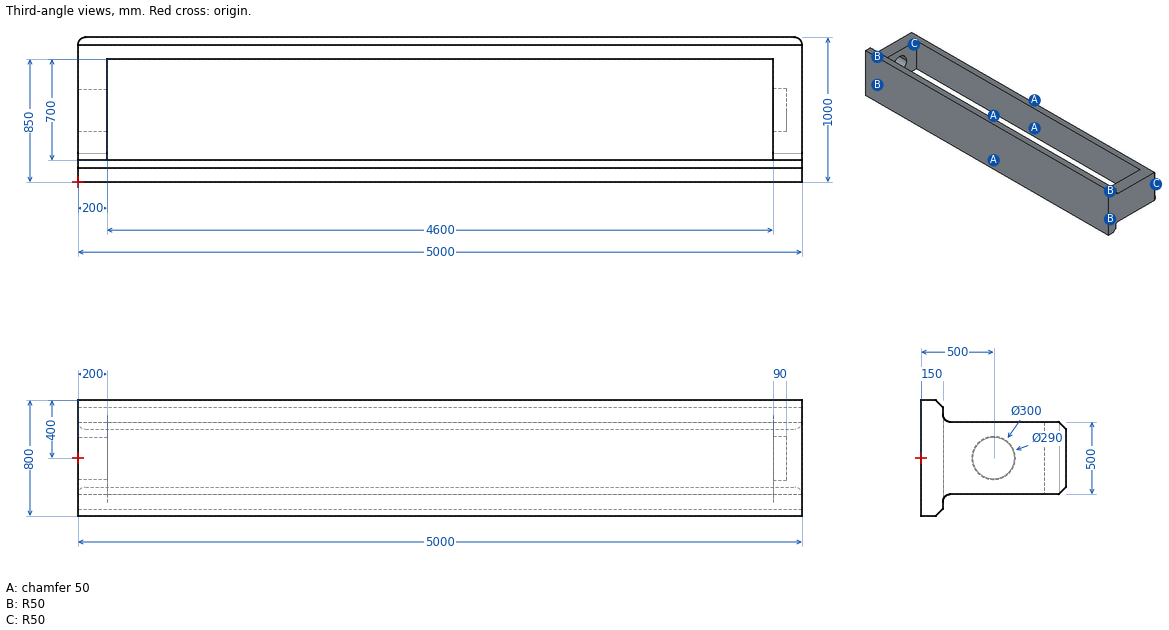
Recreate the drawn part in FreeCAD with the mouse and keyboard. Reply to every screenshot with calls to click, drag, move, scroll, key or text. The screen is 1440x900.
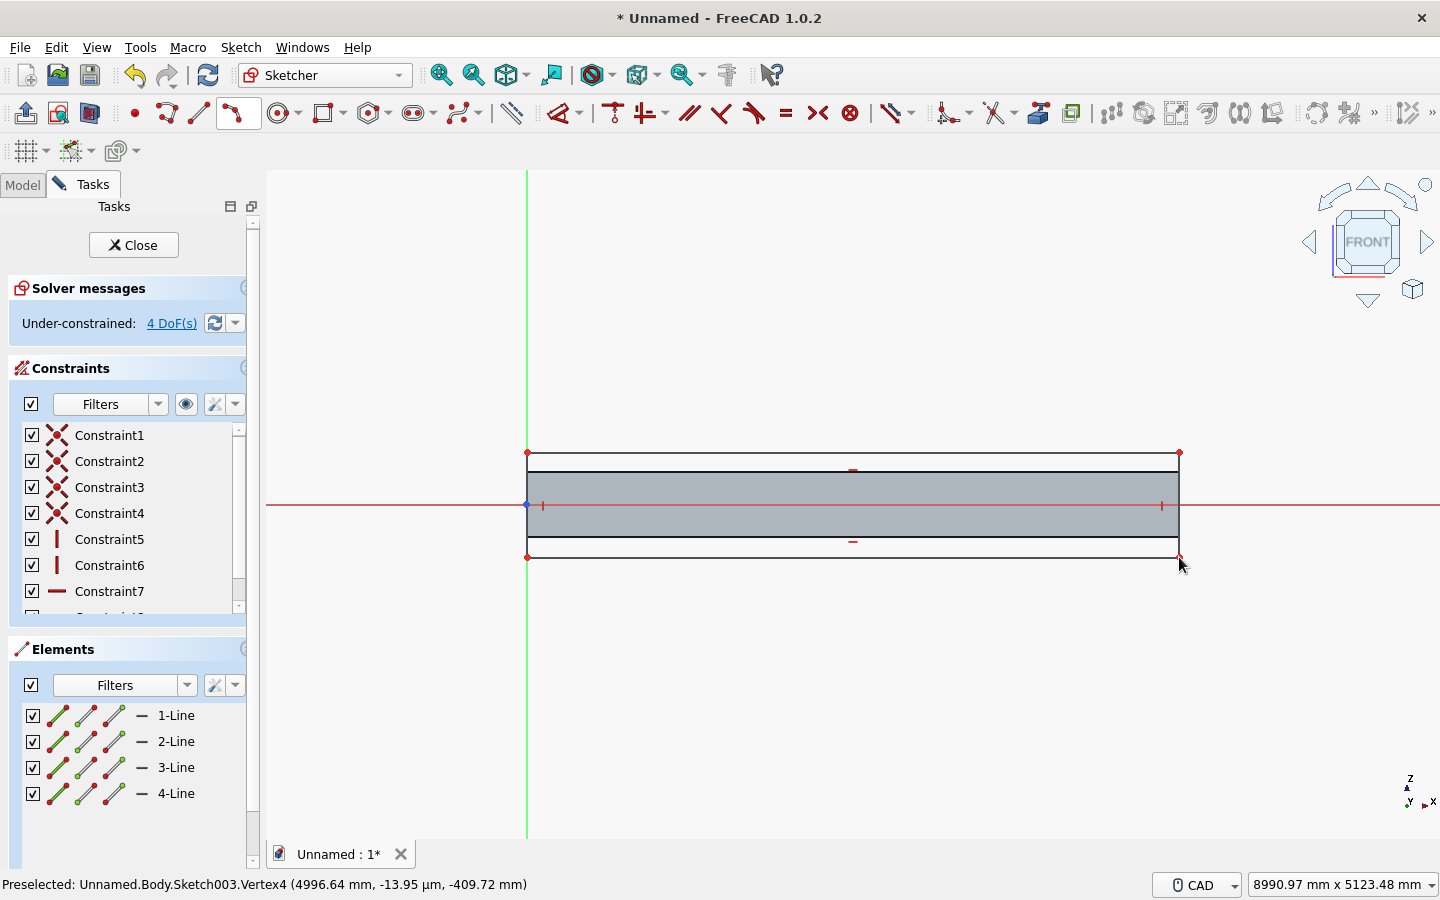
click(527, 453)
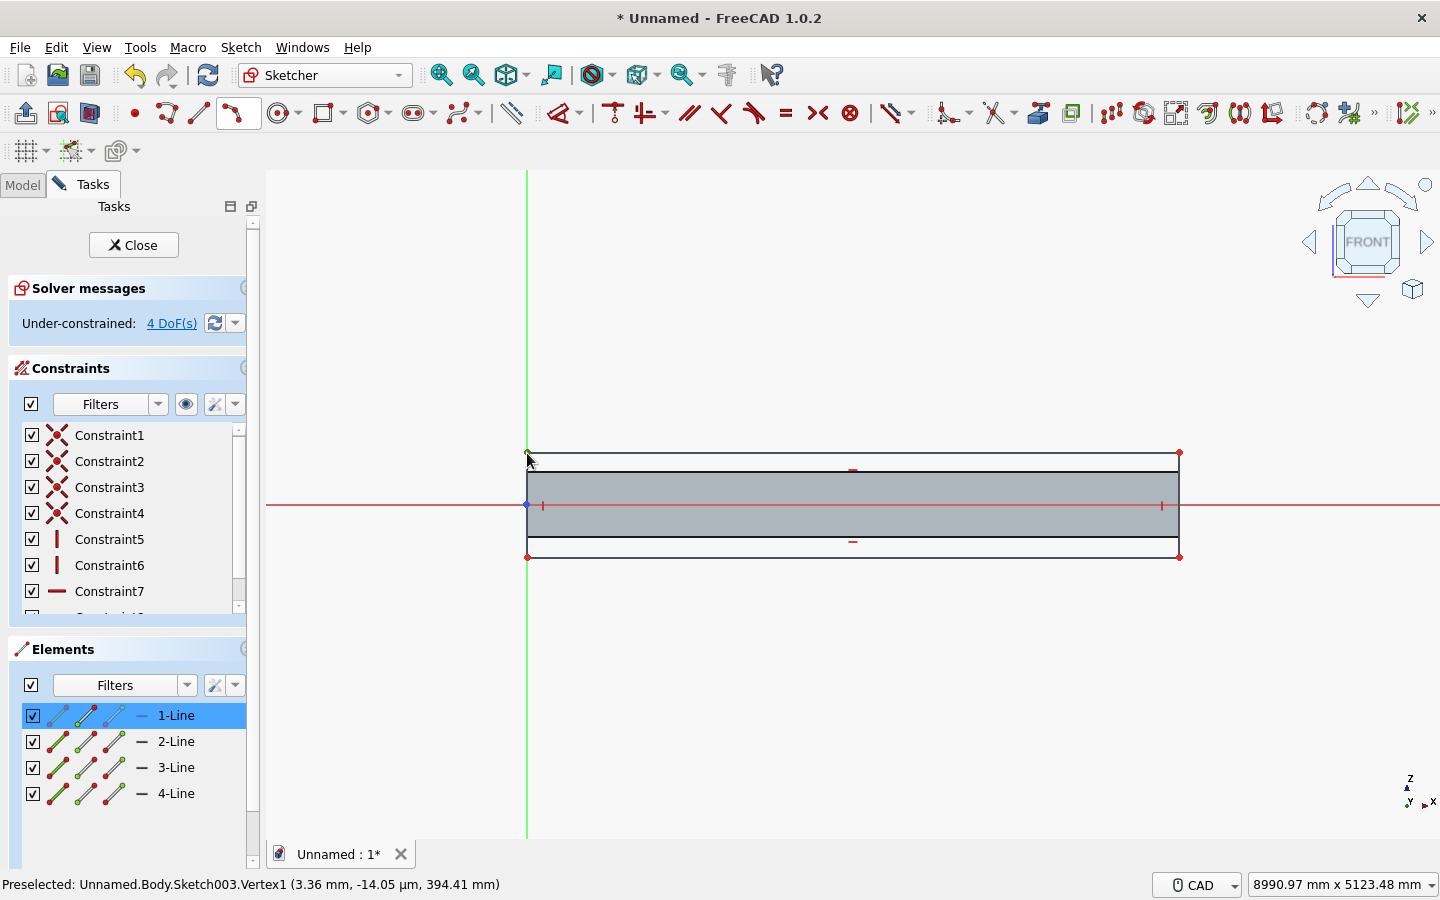
click(527, 767)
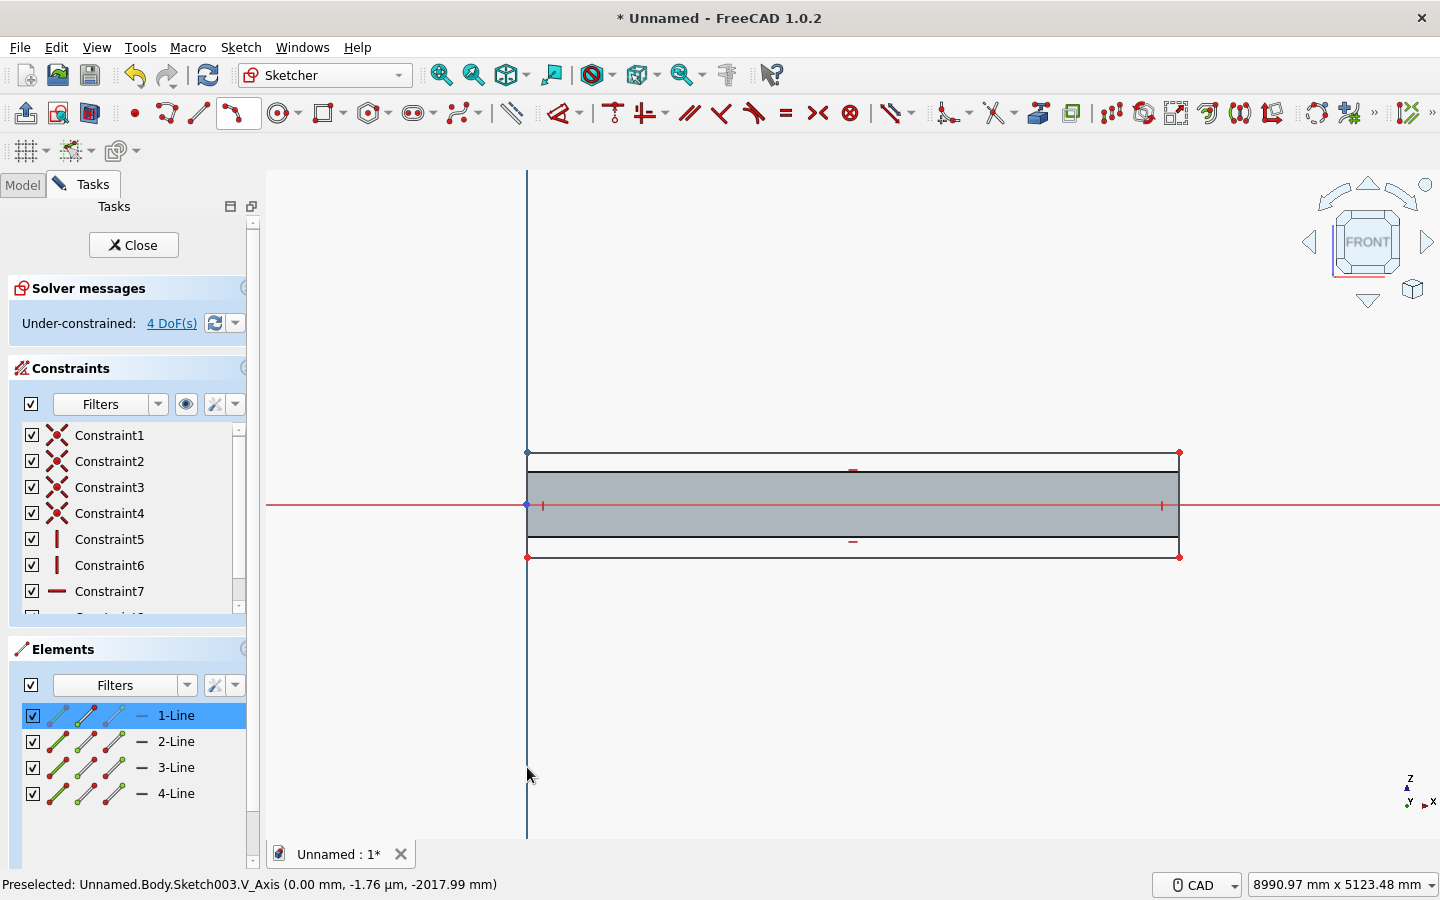
key(c)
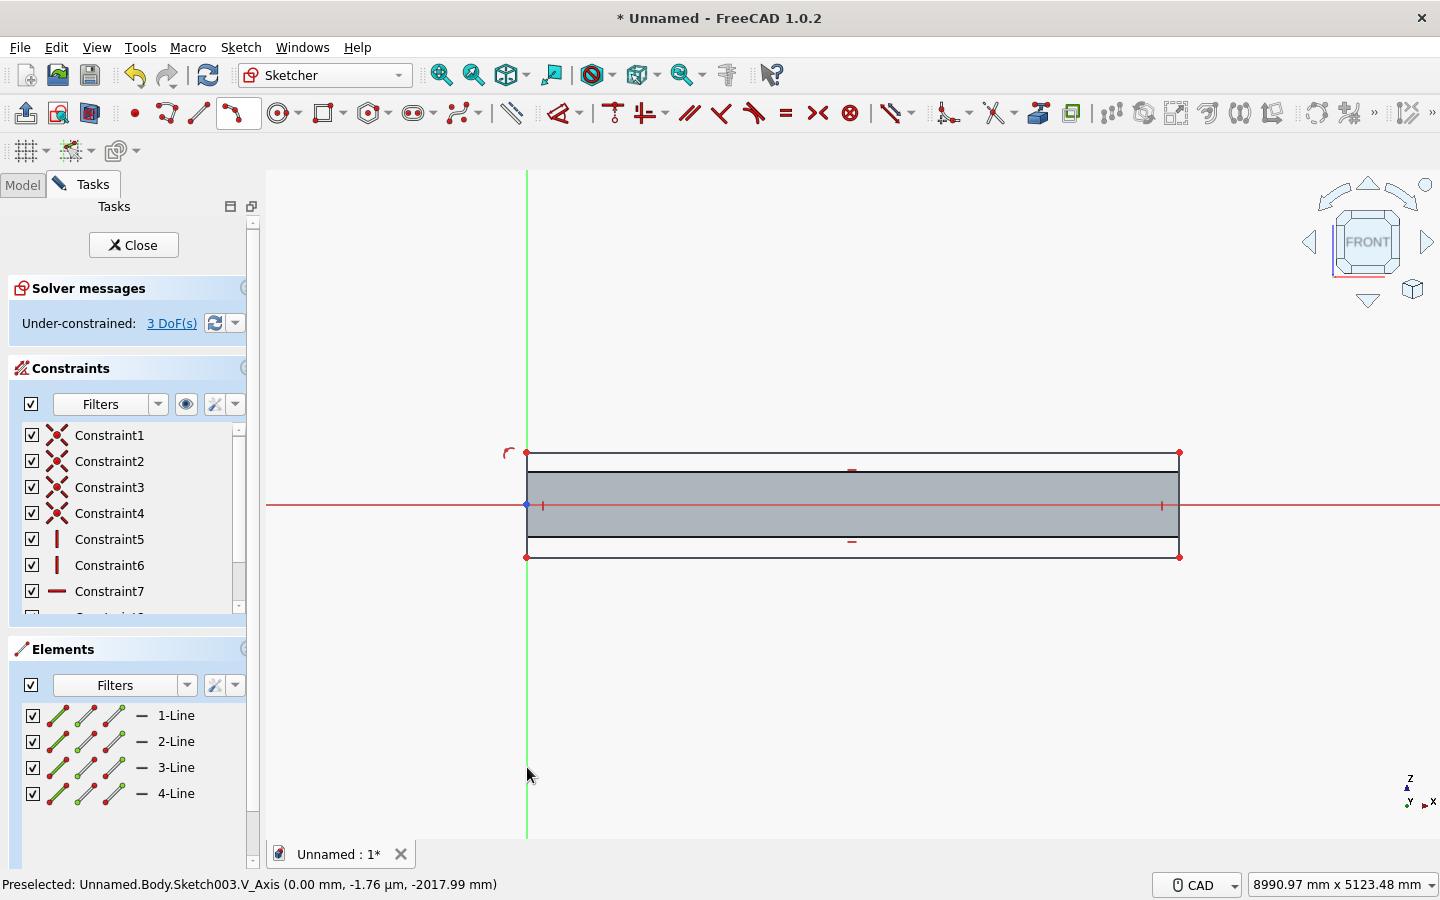
key(d)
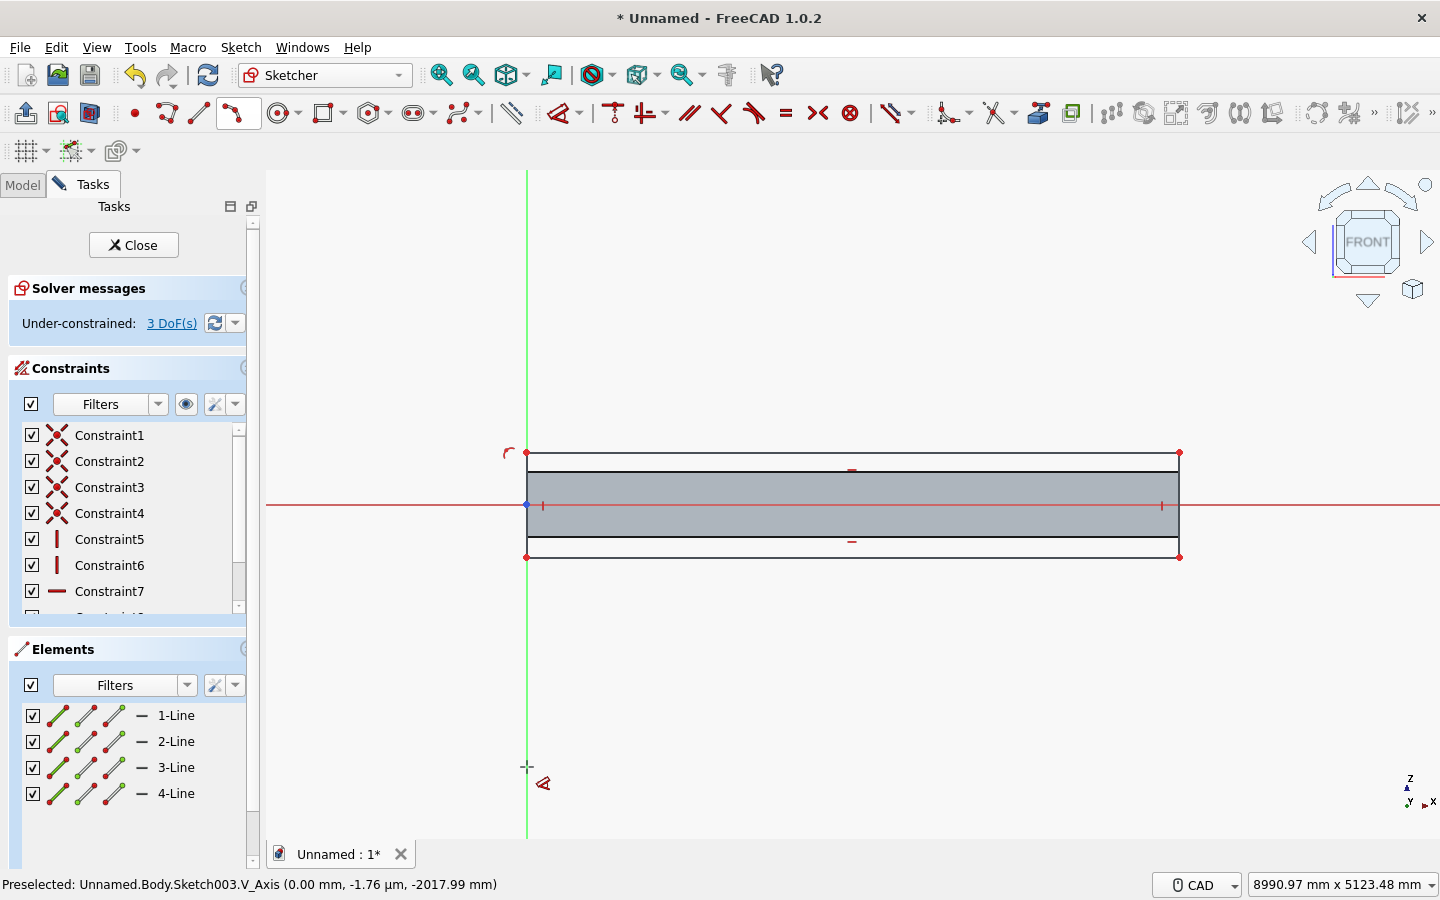
click(527, 484)
click(493, 481)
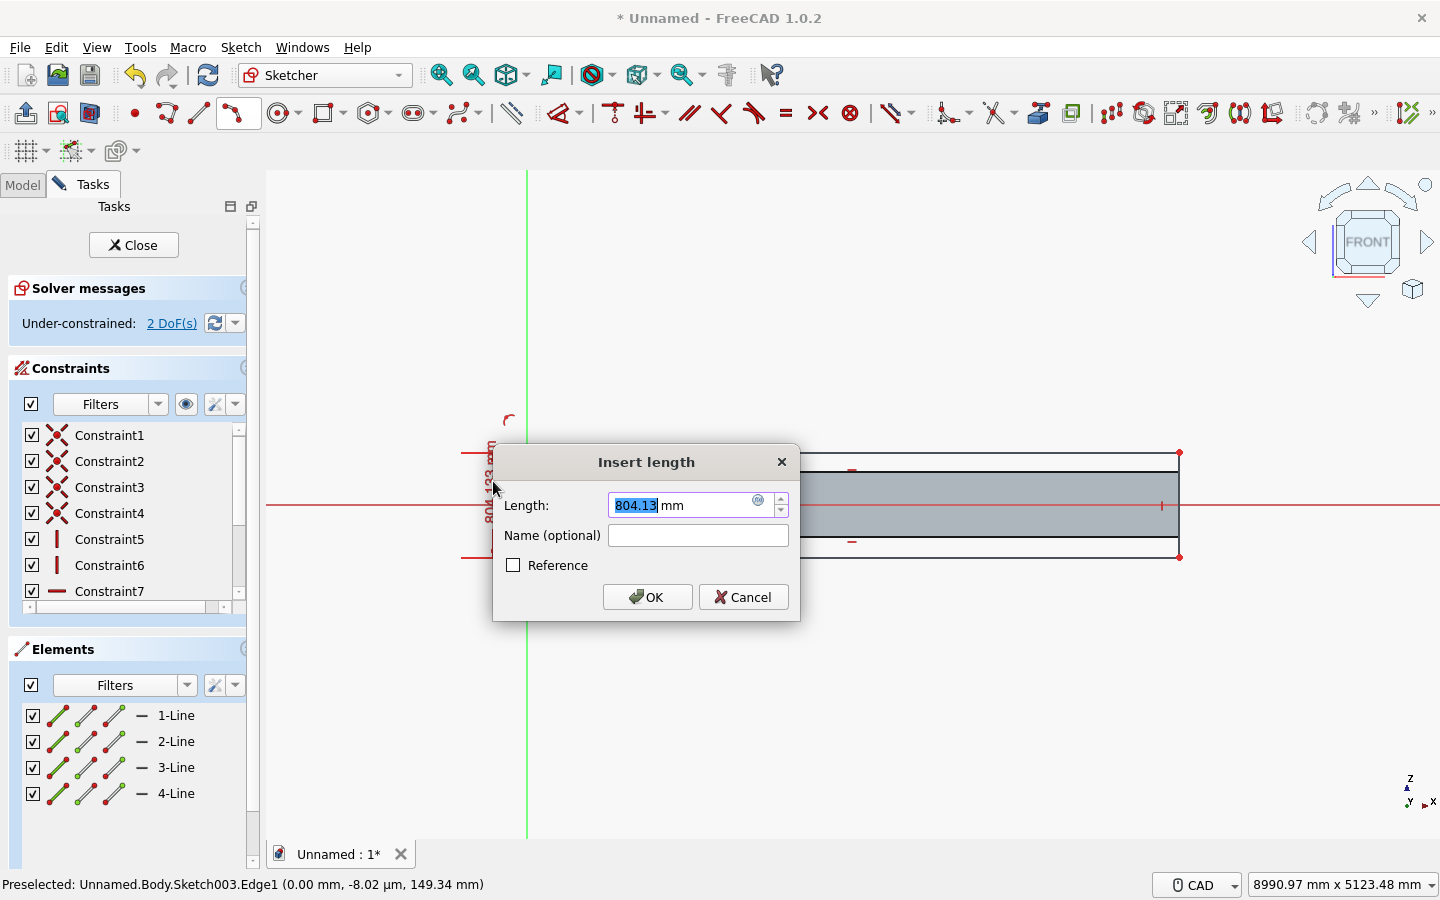
text(800)
key(Return)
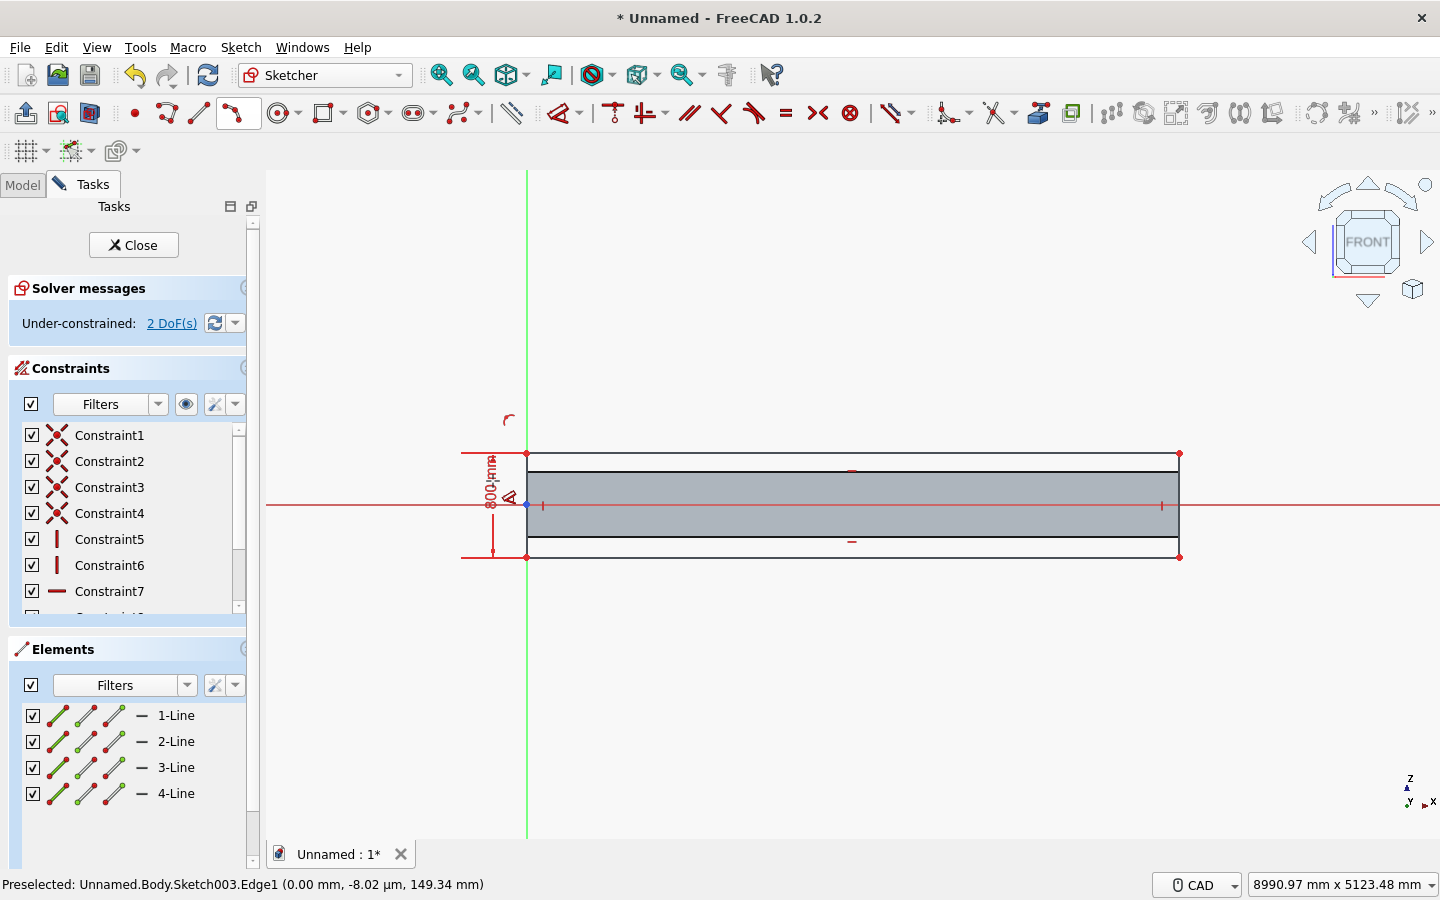
click(722, 558)
click(853, 592)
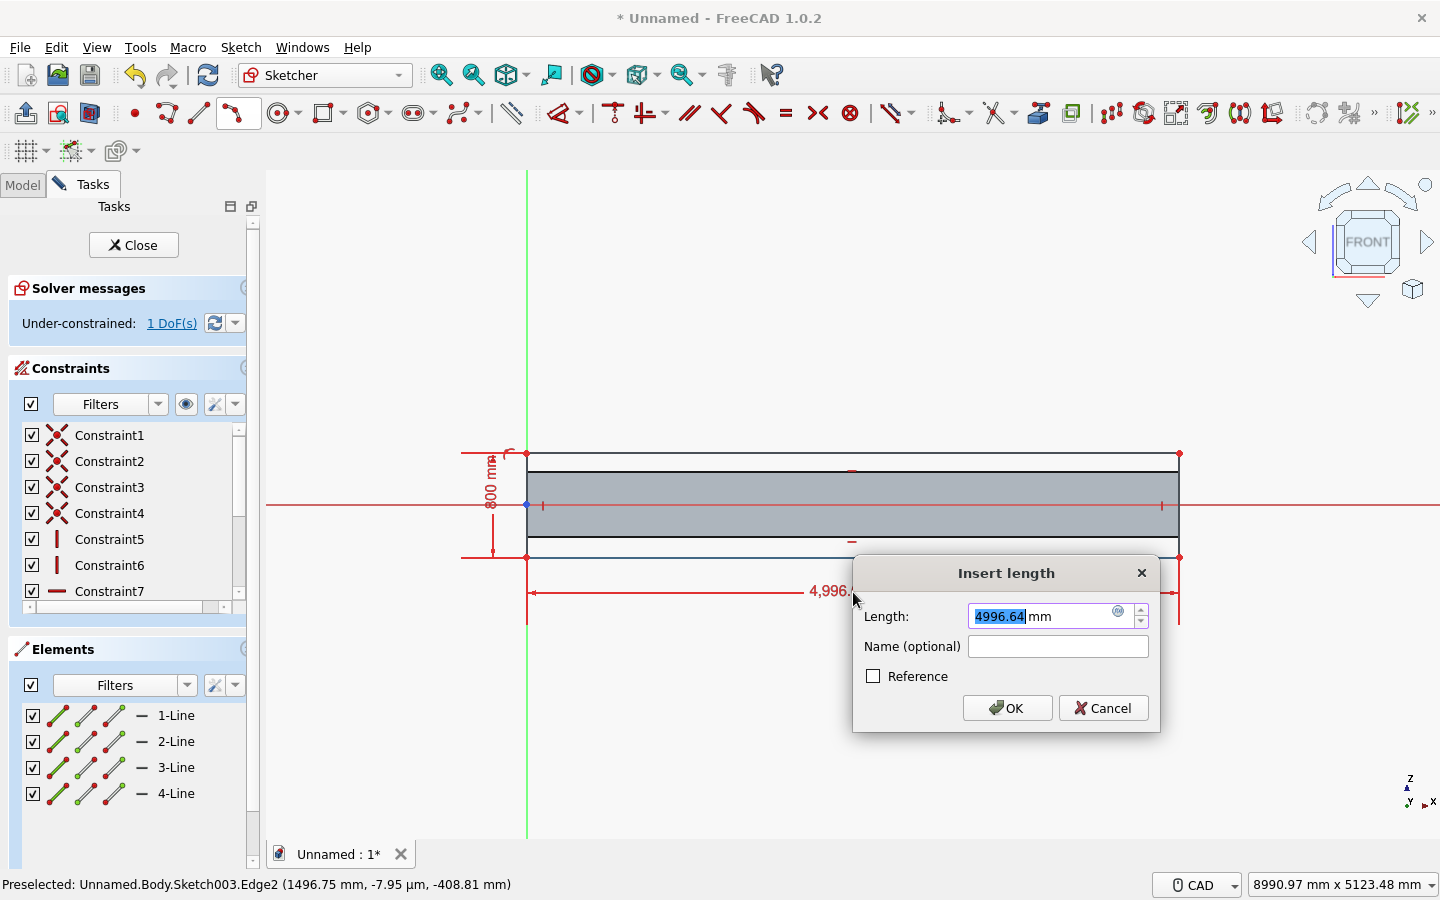
text(5000)
key(Return)